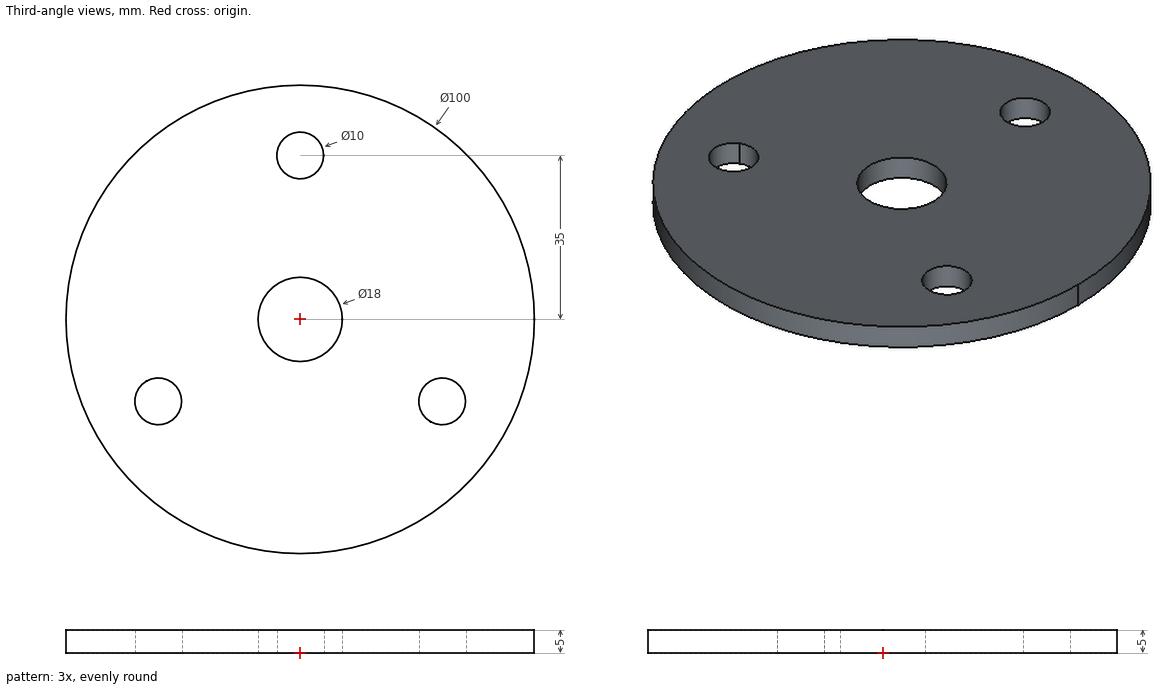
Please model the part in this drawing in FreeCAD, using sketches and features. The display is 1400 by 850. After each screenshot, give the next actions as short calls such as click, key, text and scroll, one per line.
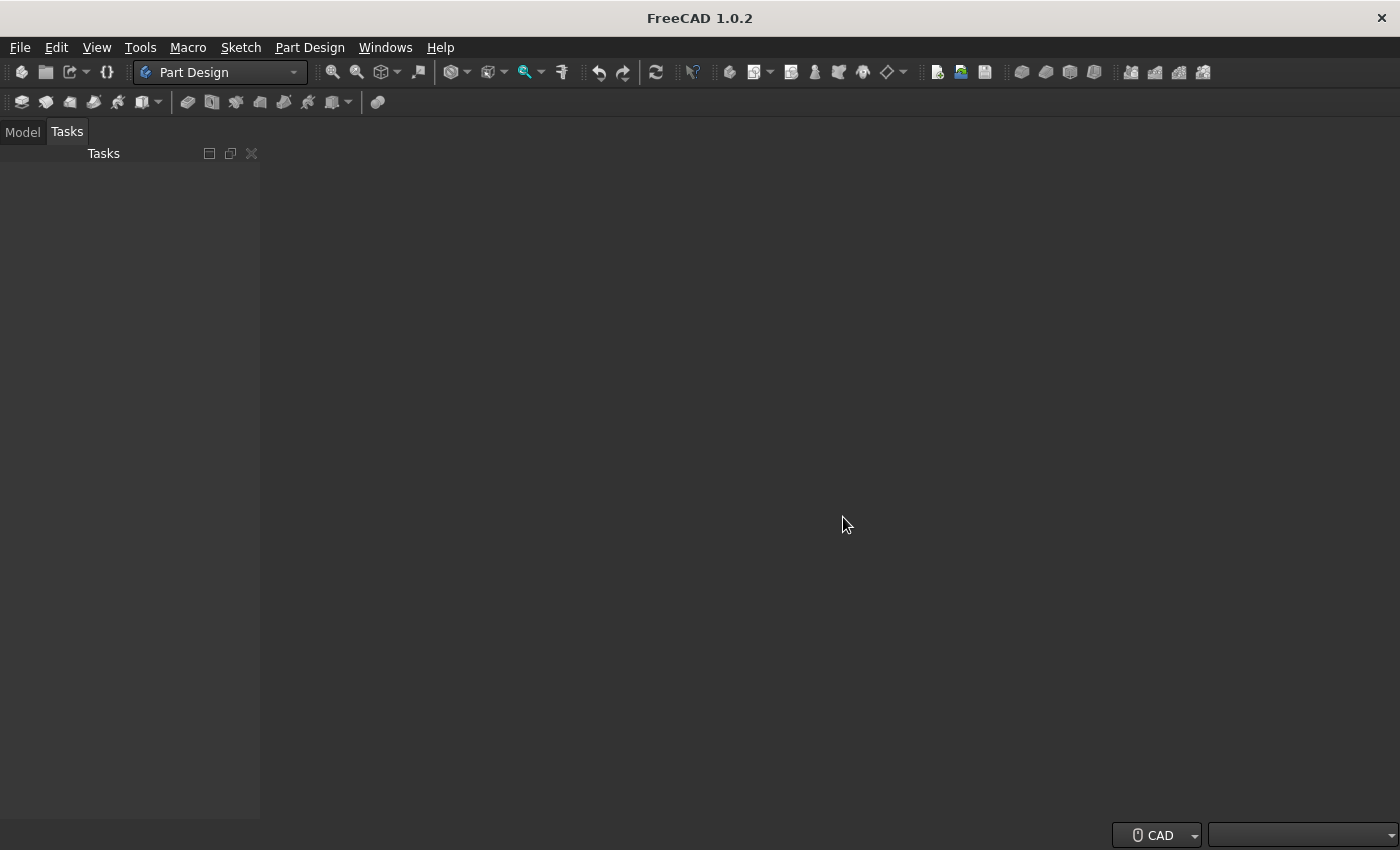
click(938, 72)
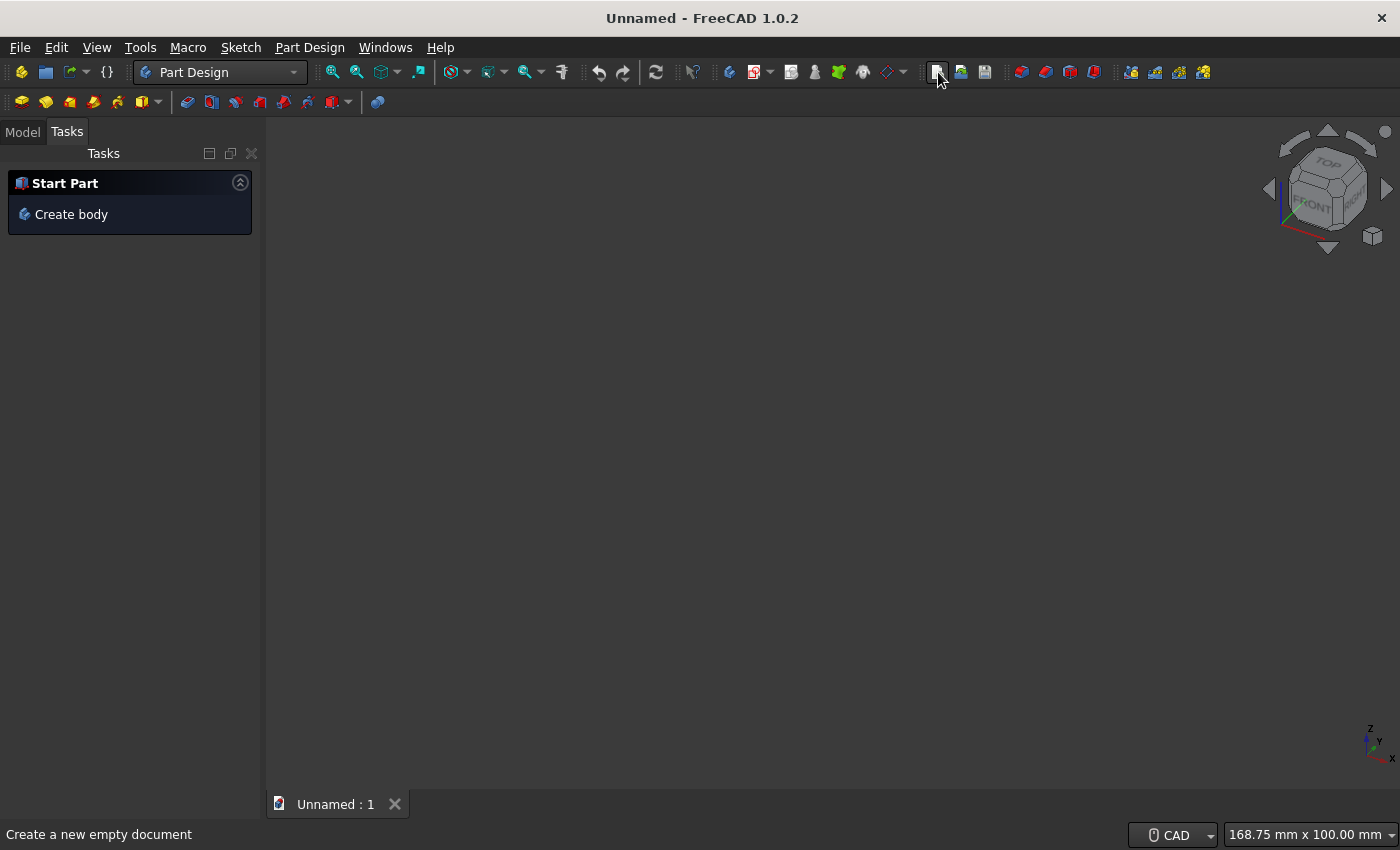
click(754, 72)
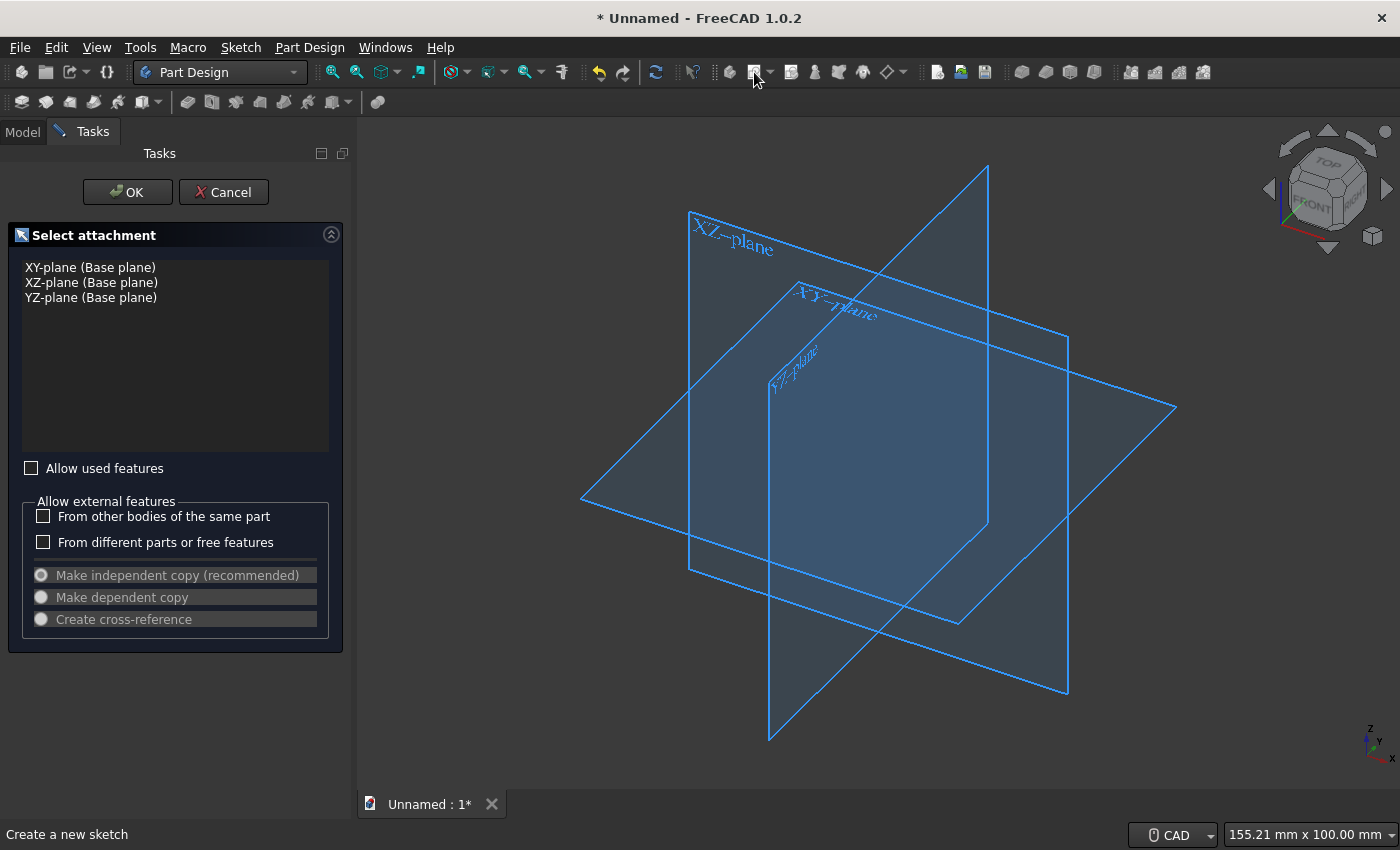
click(82, 268)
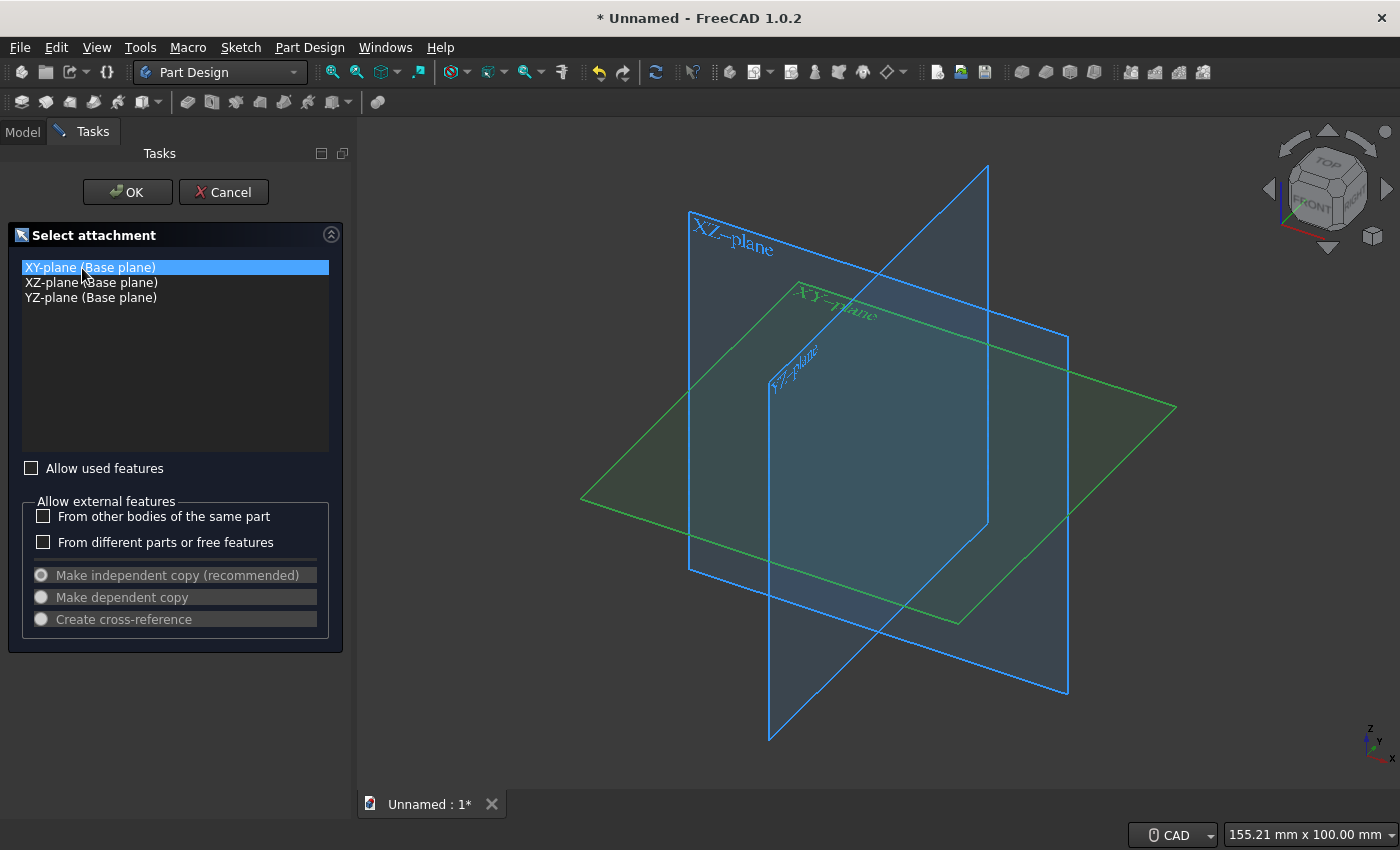
click(128, 192)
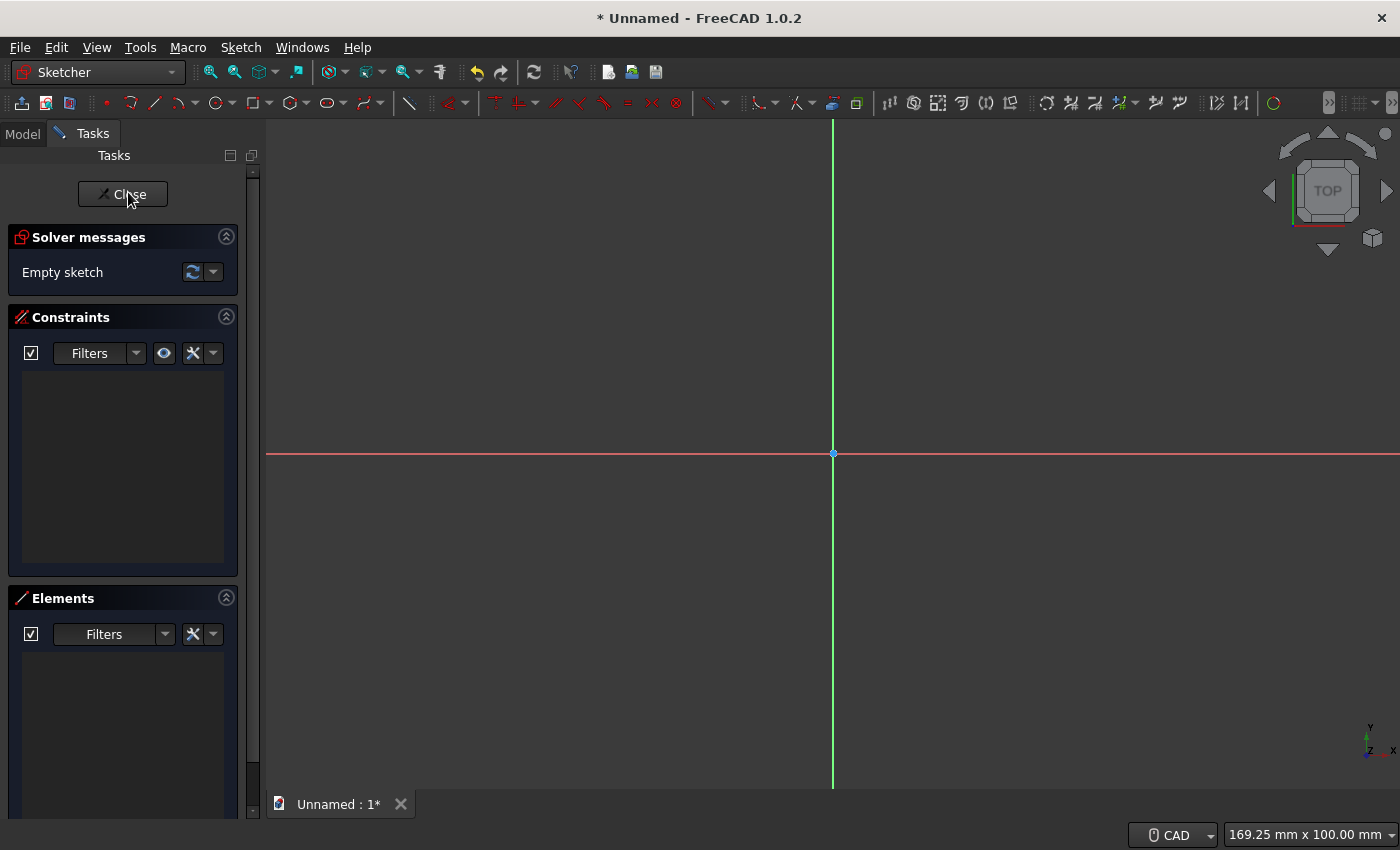
scroll(625, 454, down, 2)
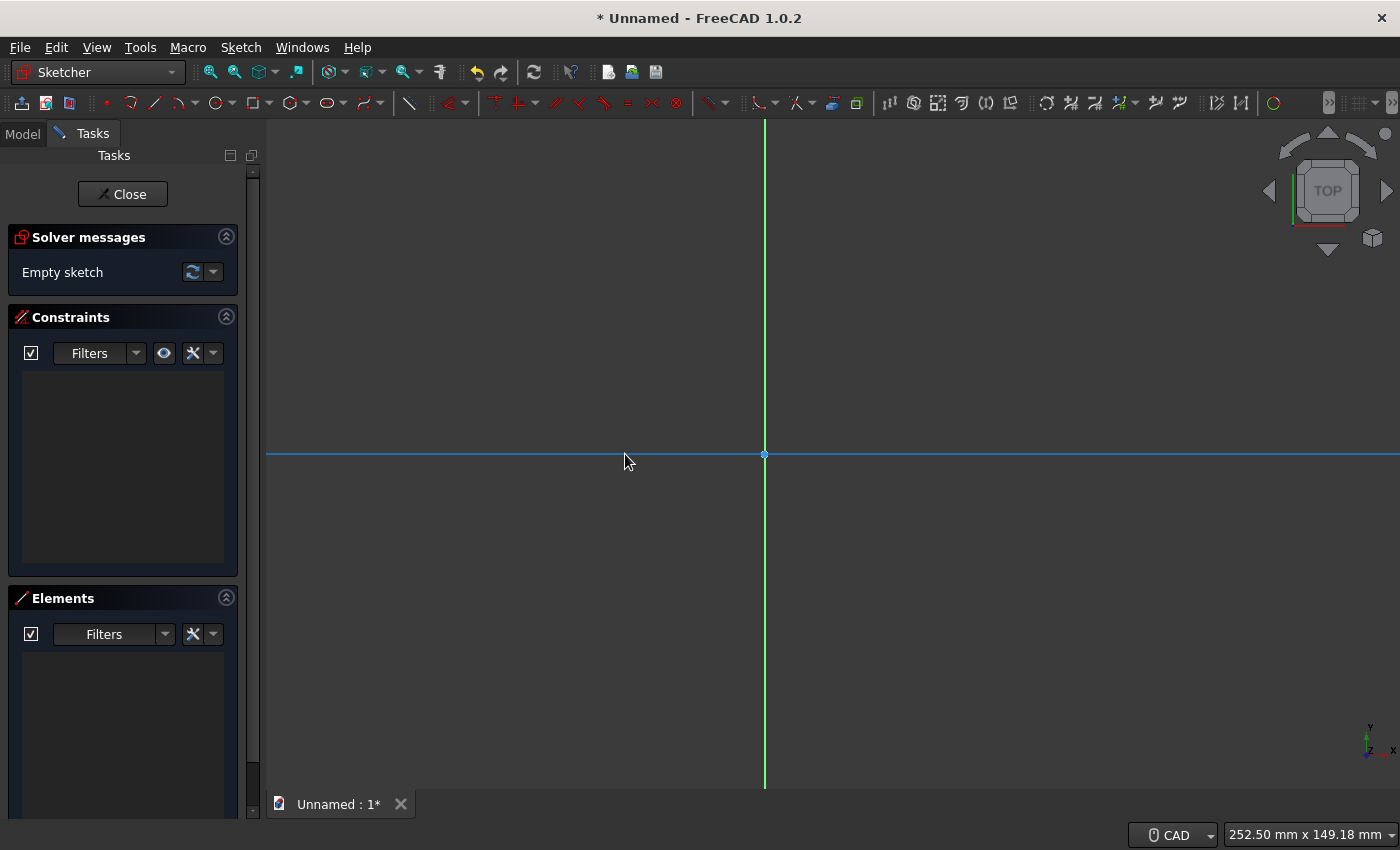
click(216, 104)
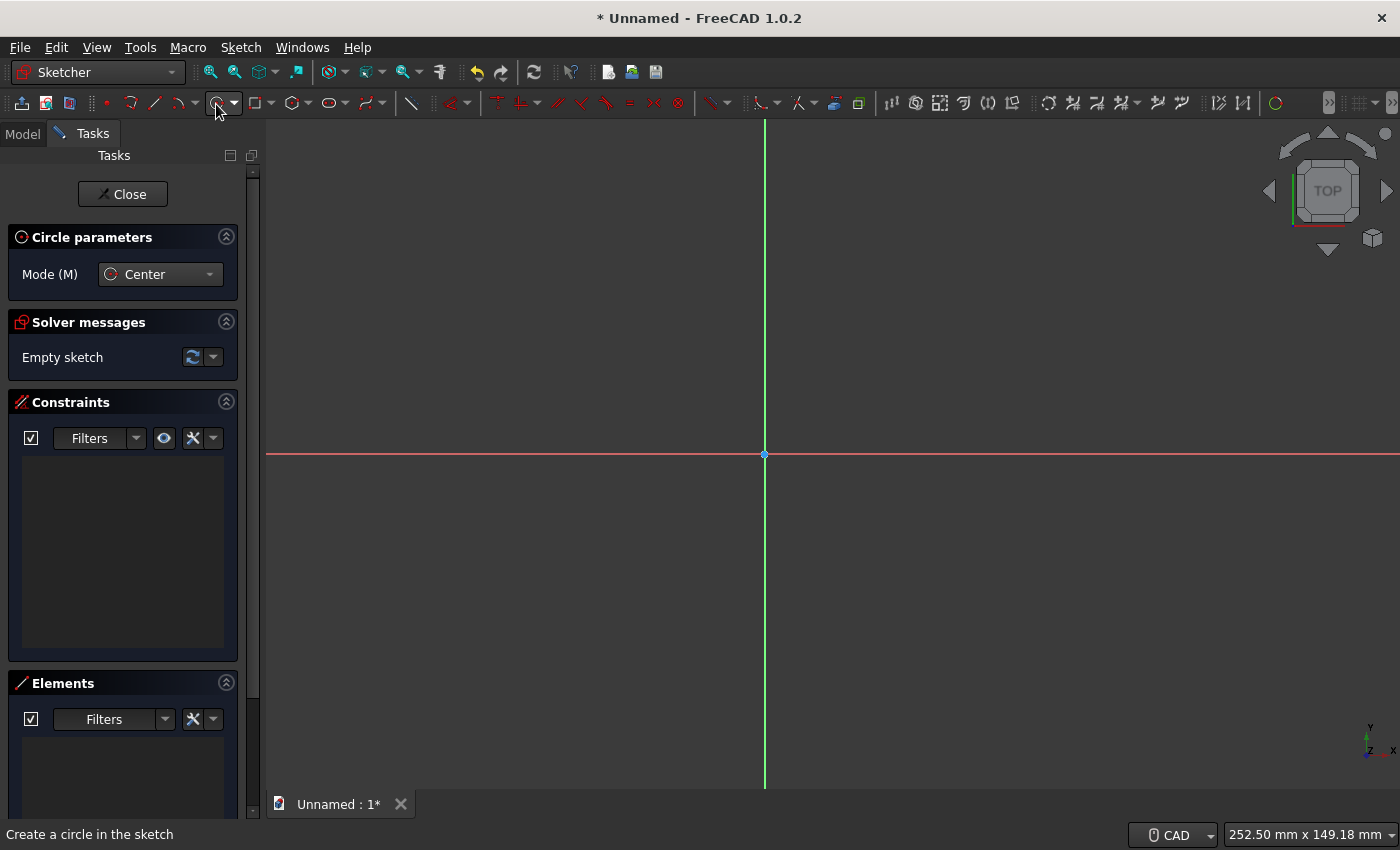
click(765, 454)
click(923, 295)
key(Escape)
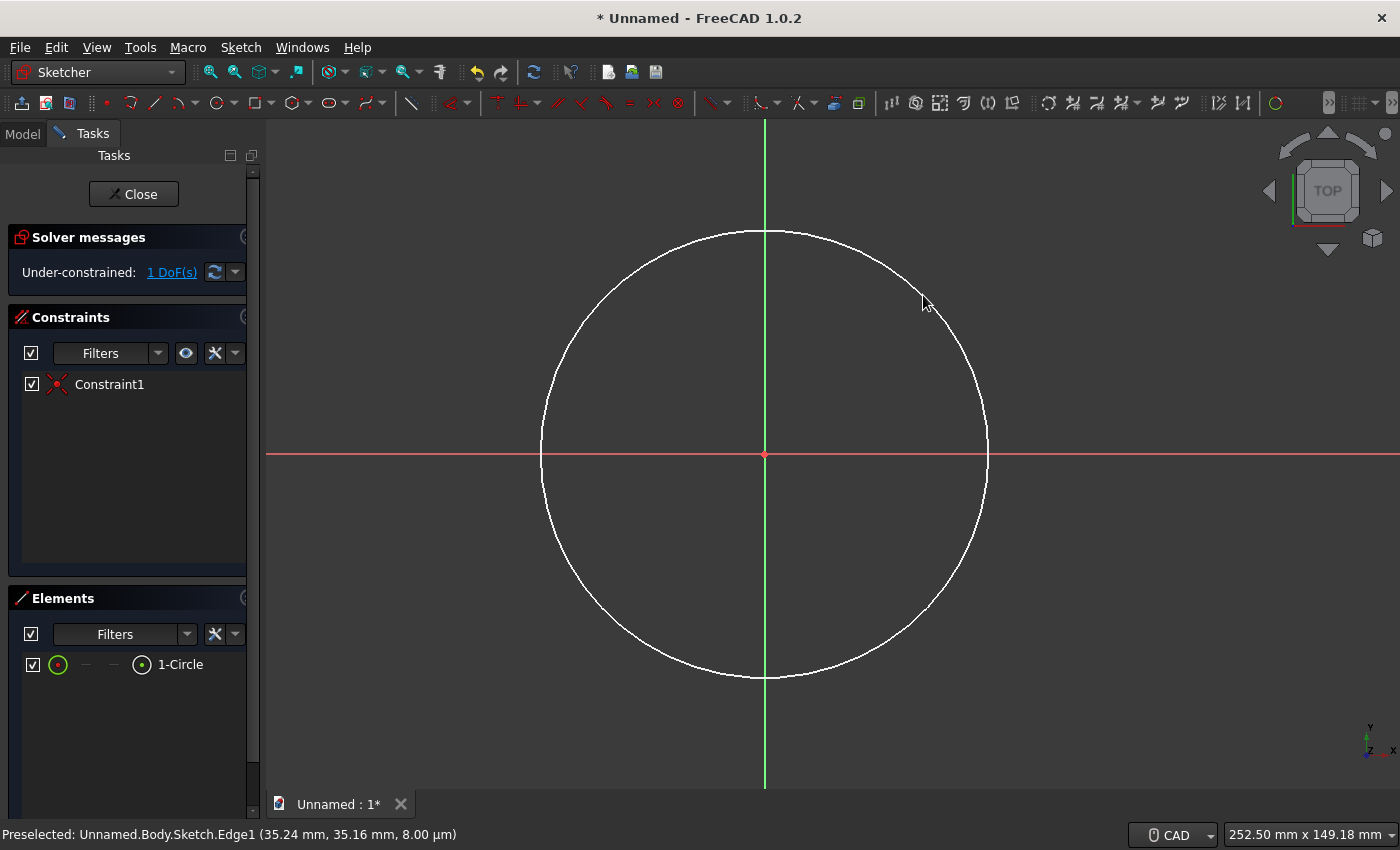
click(450, 104)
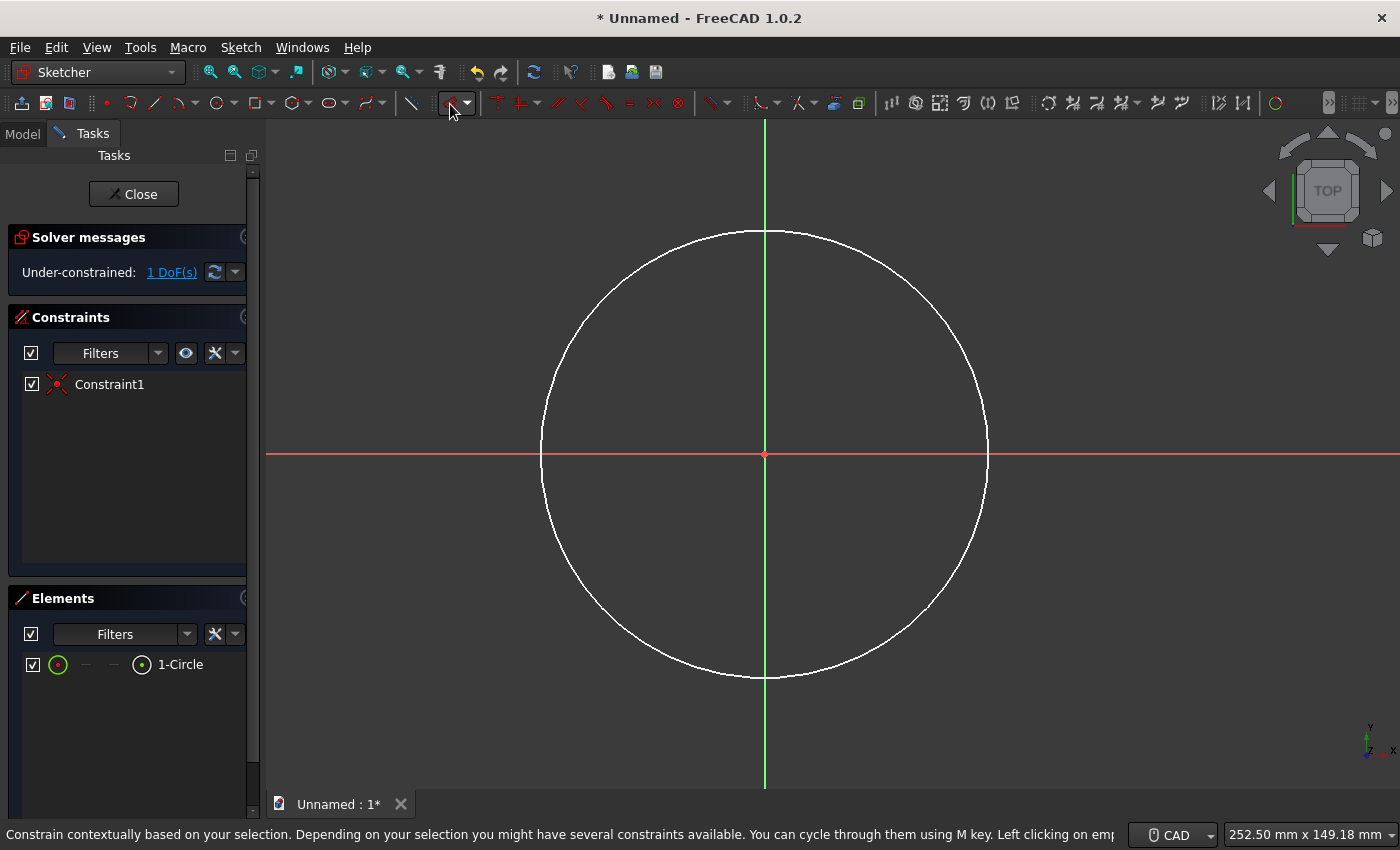
click(922, 295)
click(945, 272)